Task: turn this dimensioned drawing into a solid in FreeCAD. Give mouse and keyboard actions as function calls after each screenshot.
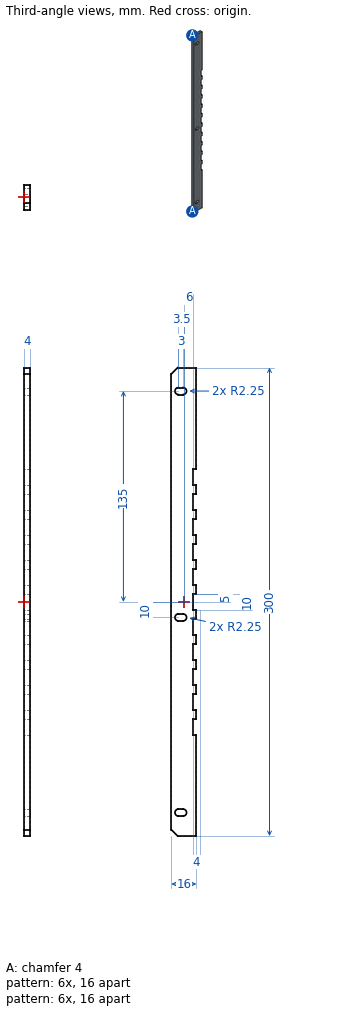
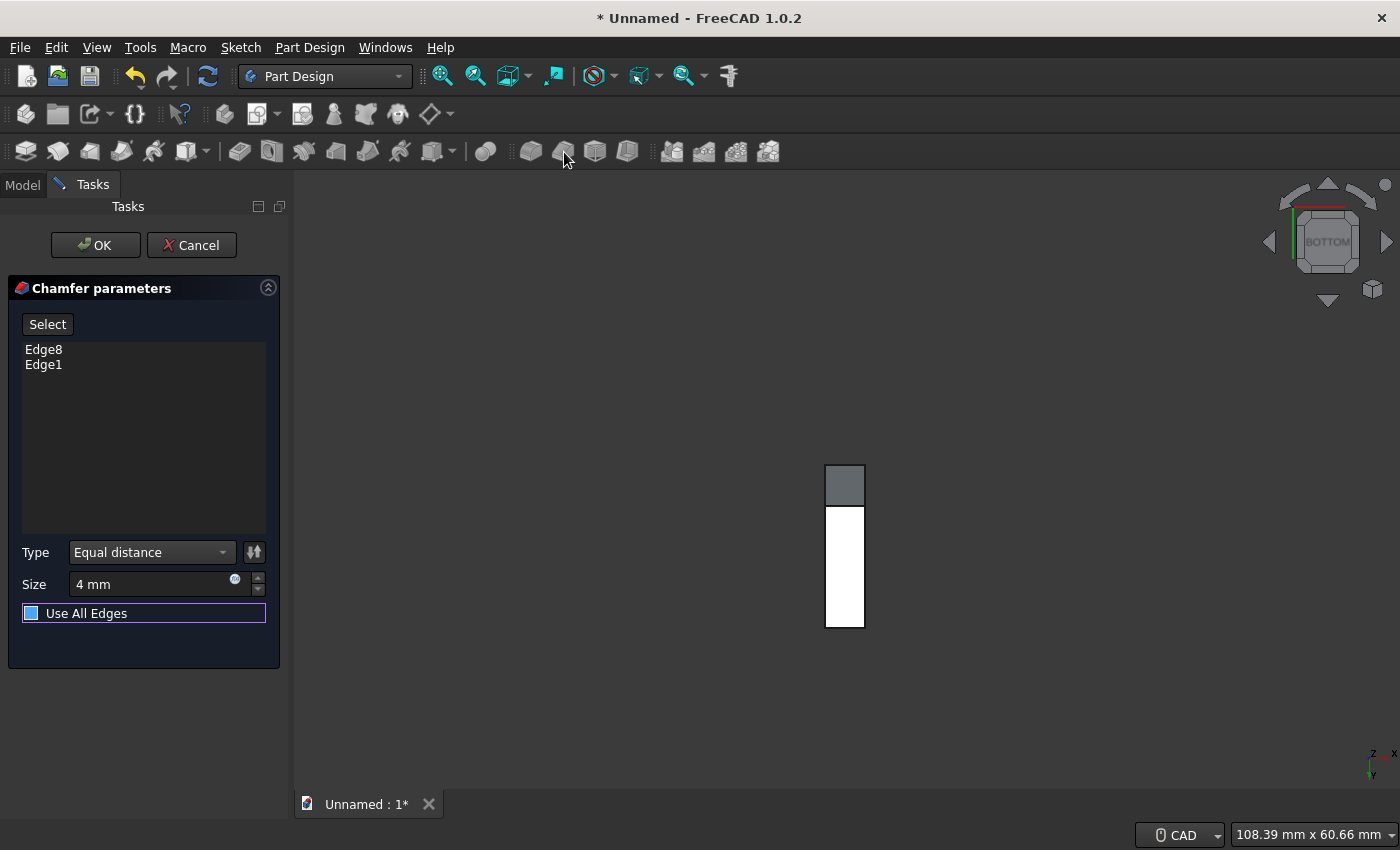
click(96, 245)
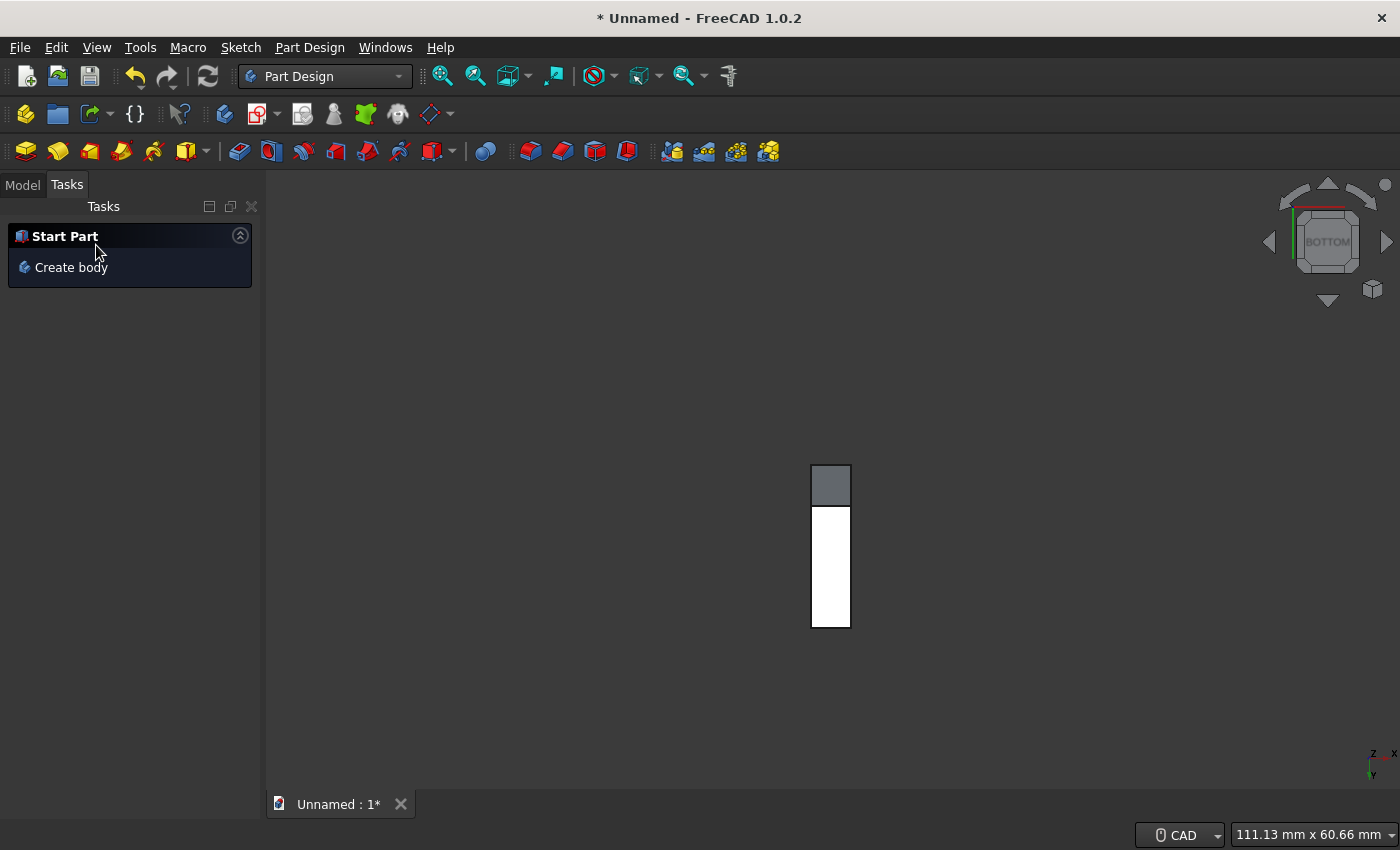
key(v)
key(f)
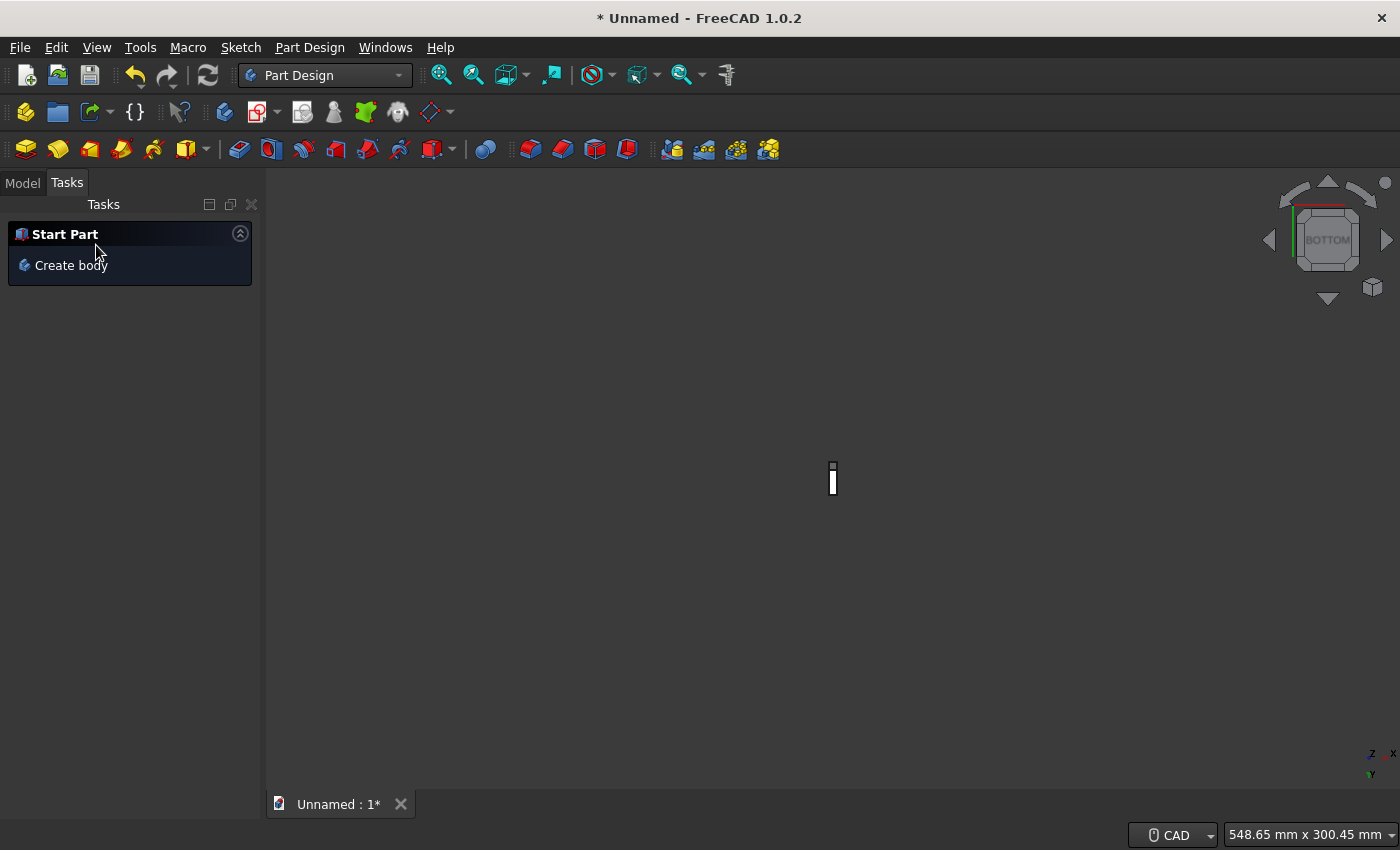
key(0)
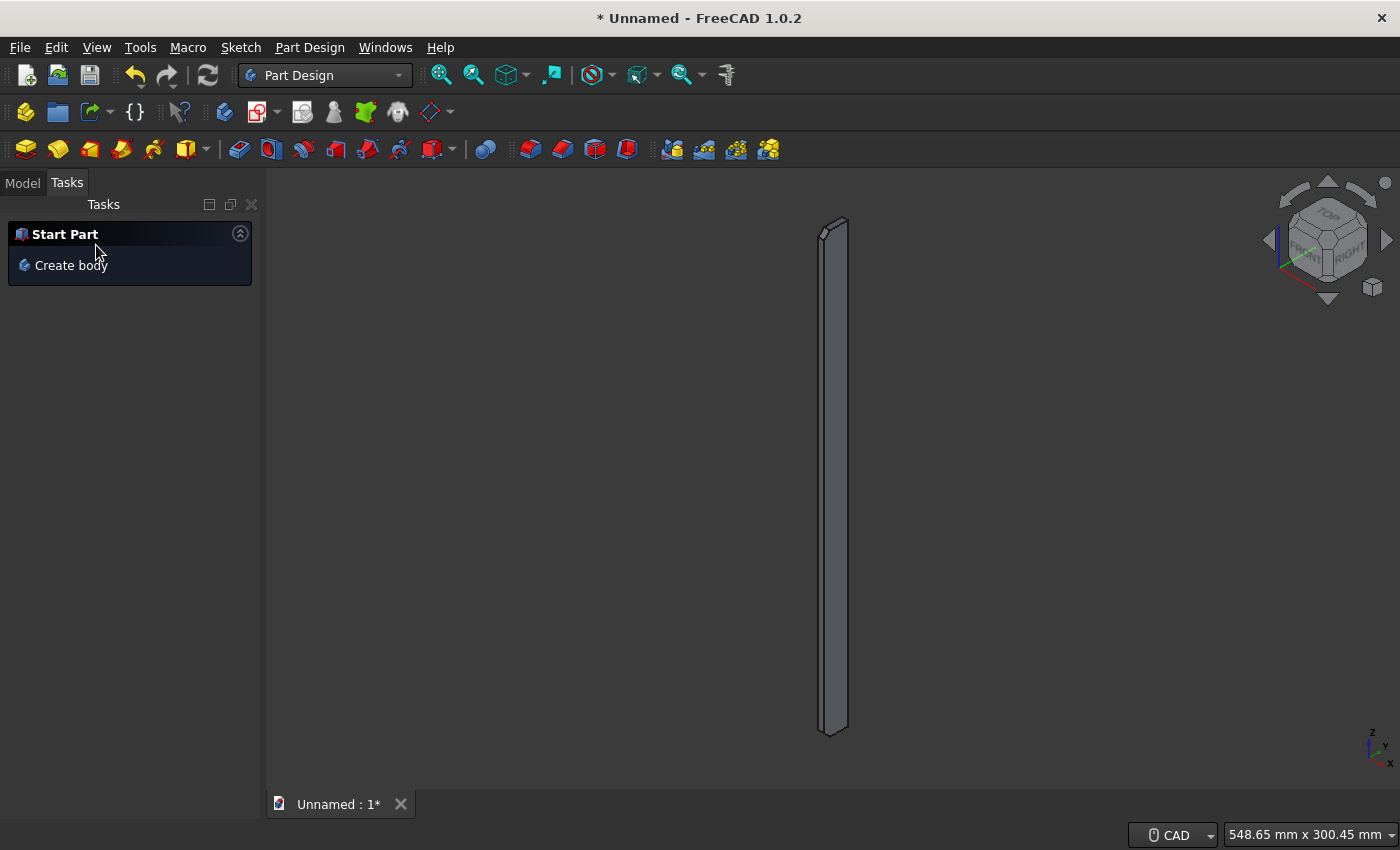
click(836, 624)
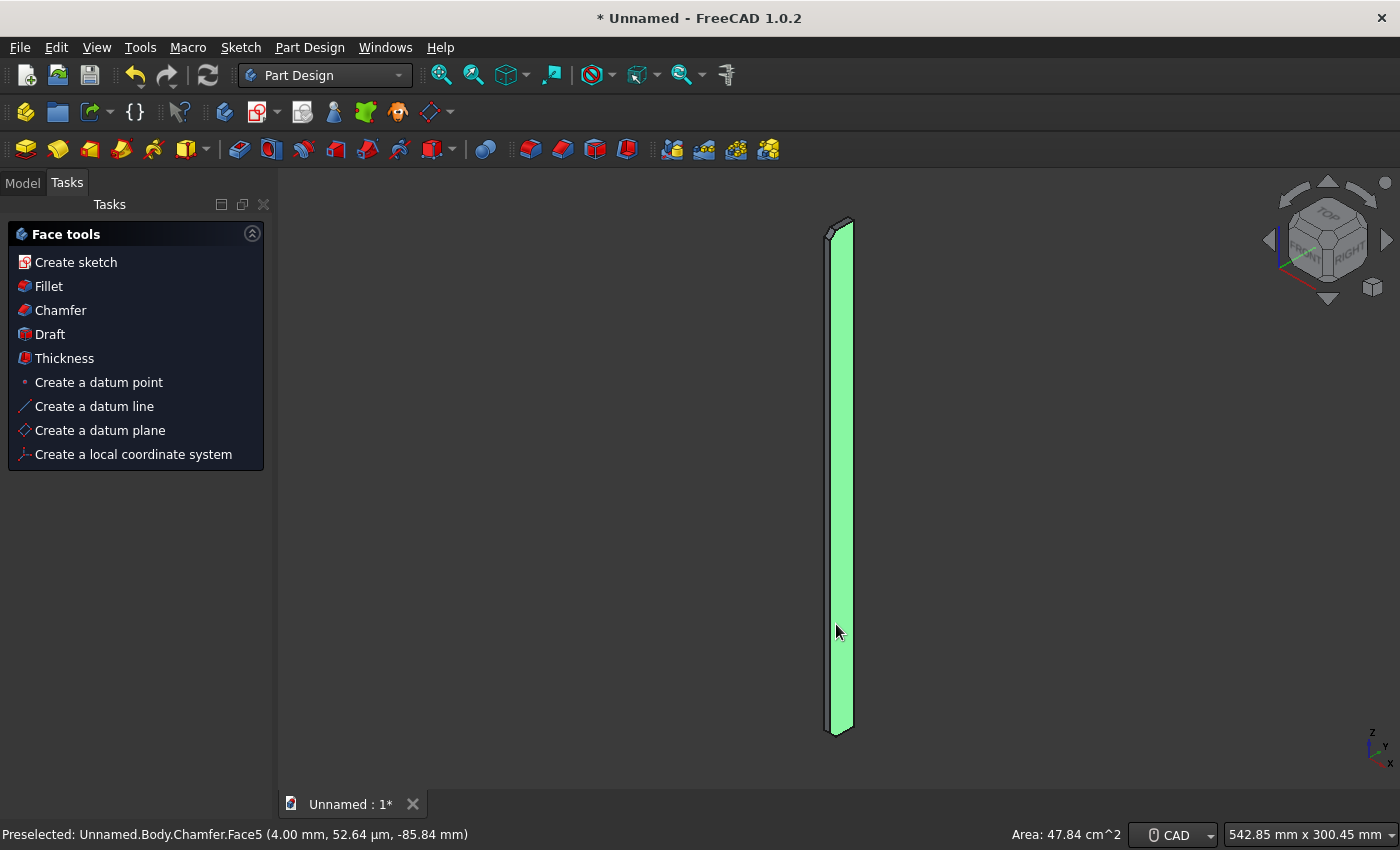
click(258, 112)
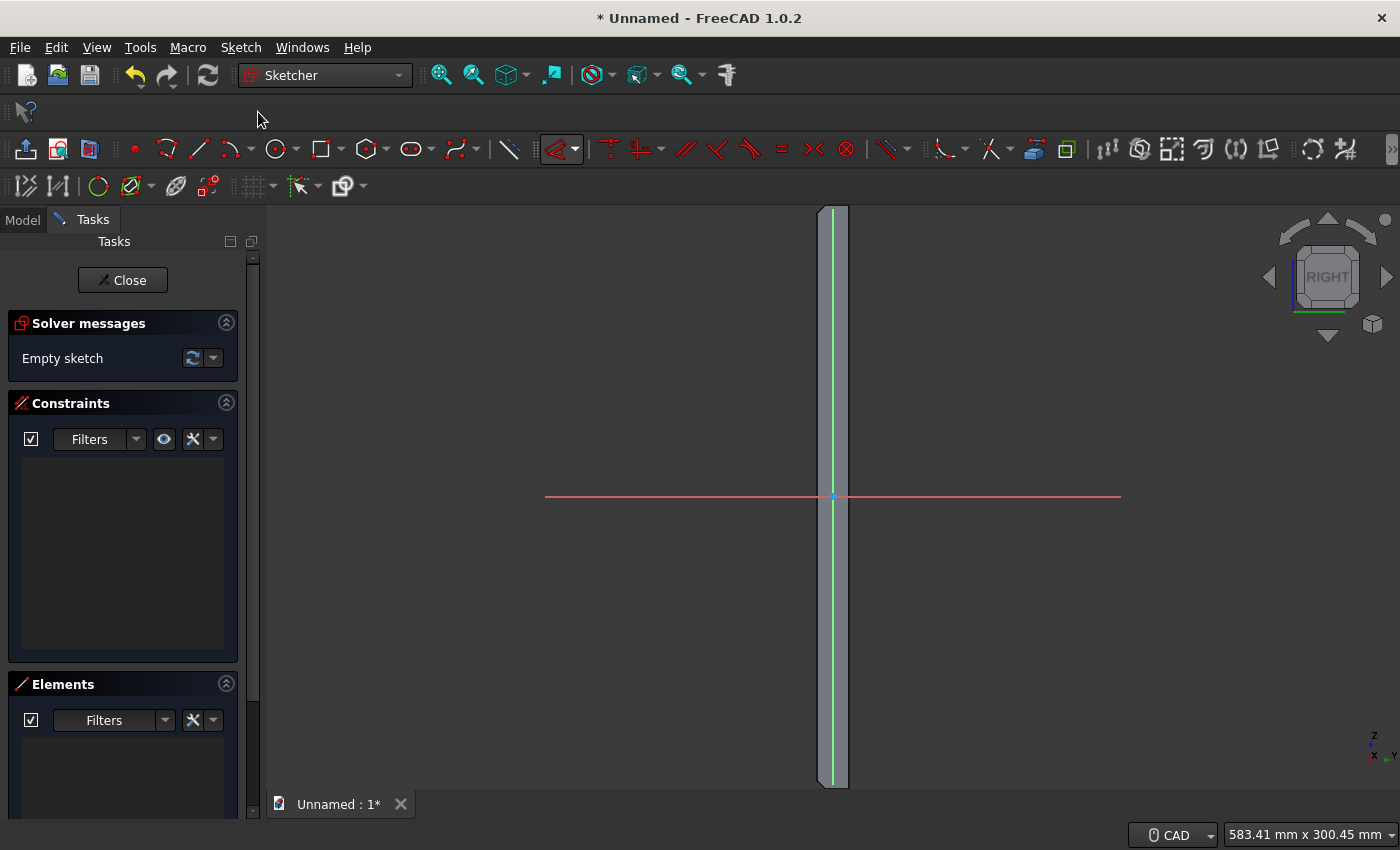
scroll(764, 497, down, 5)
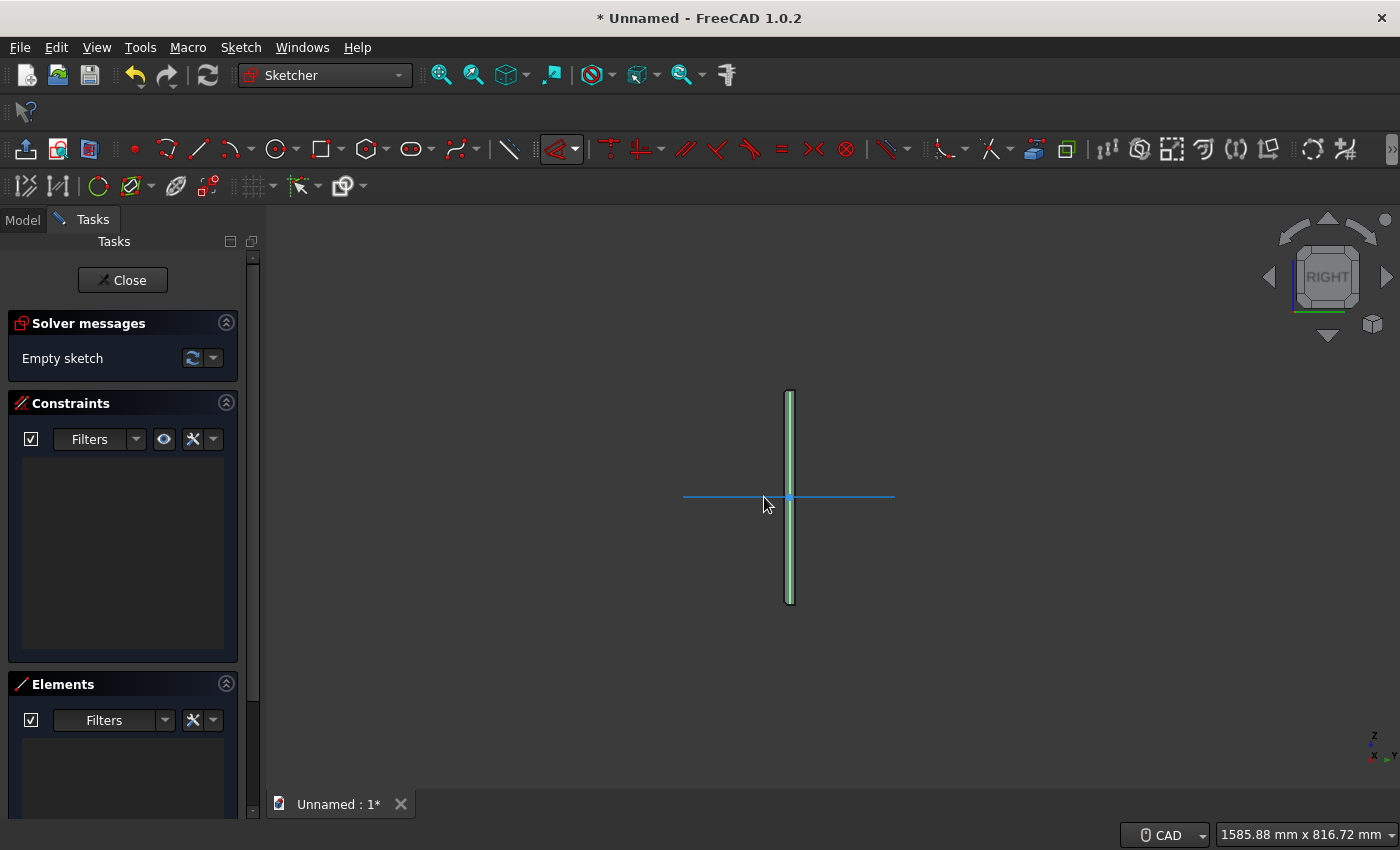
scroll(789, 396, up, 15)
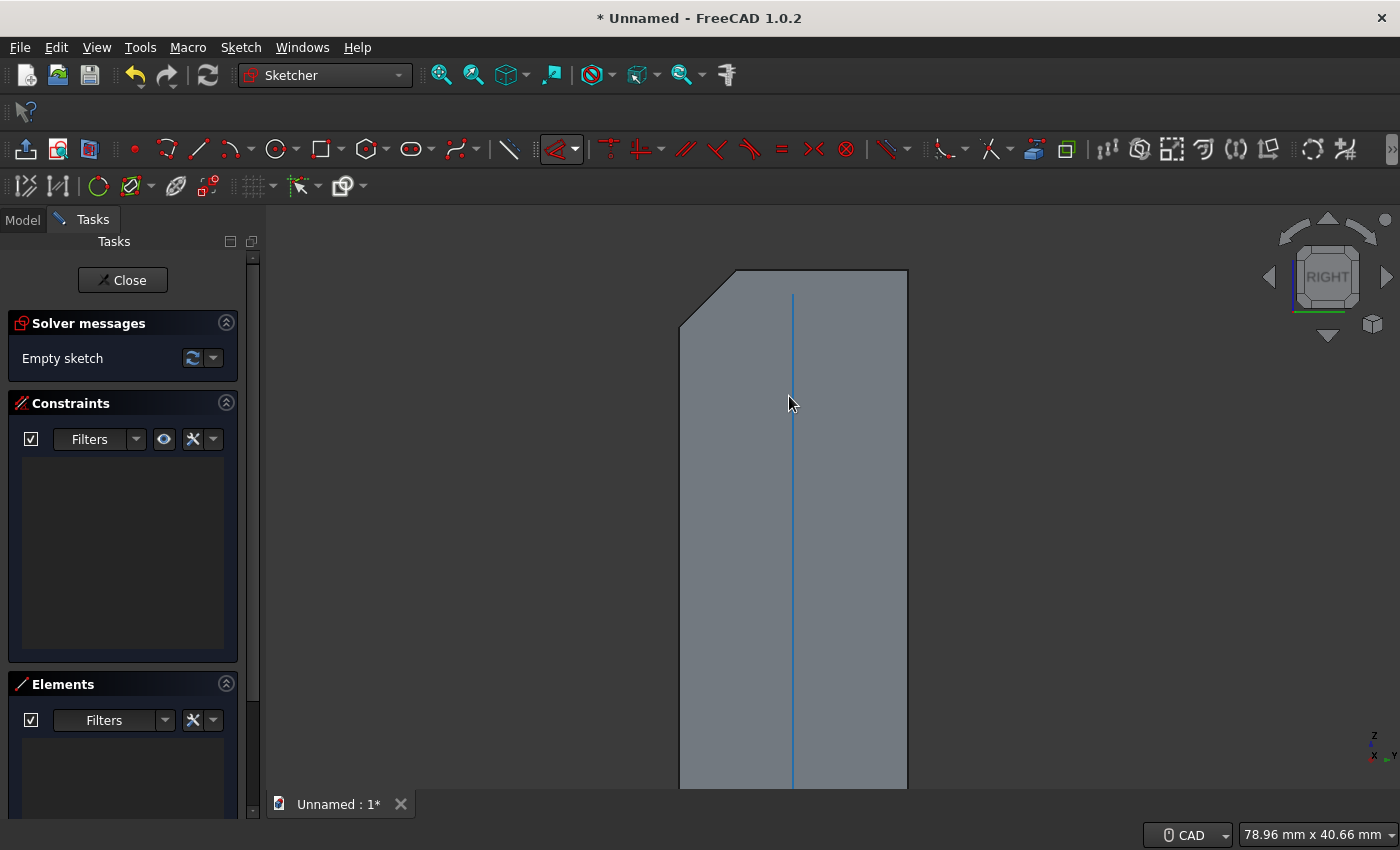
scroll(765, 484, up, 9)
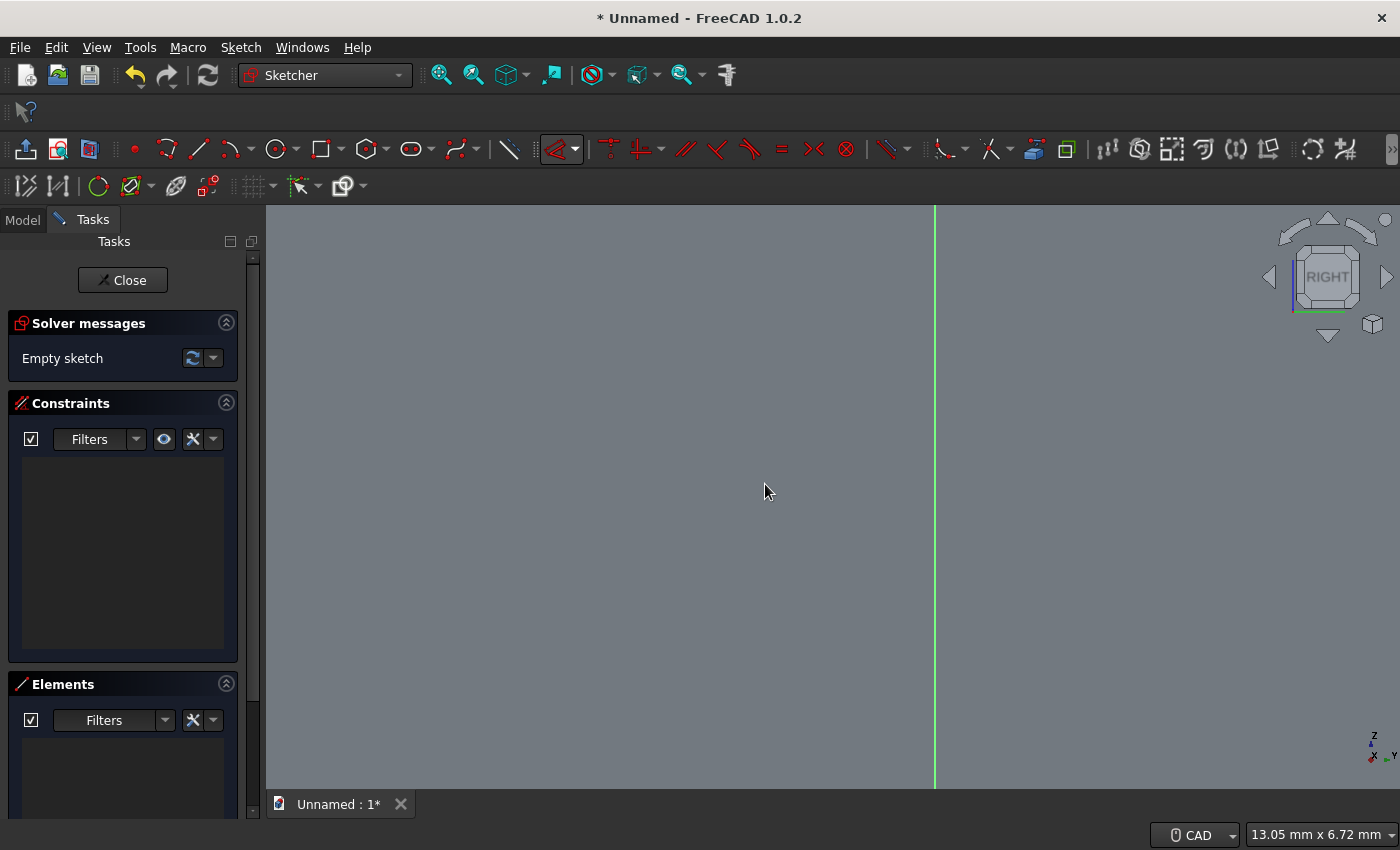
key(g)
key(s)